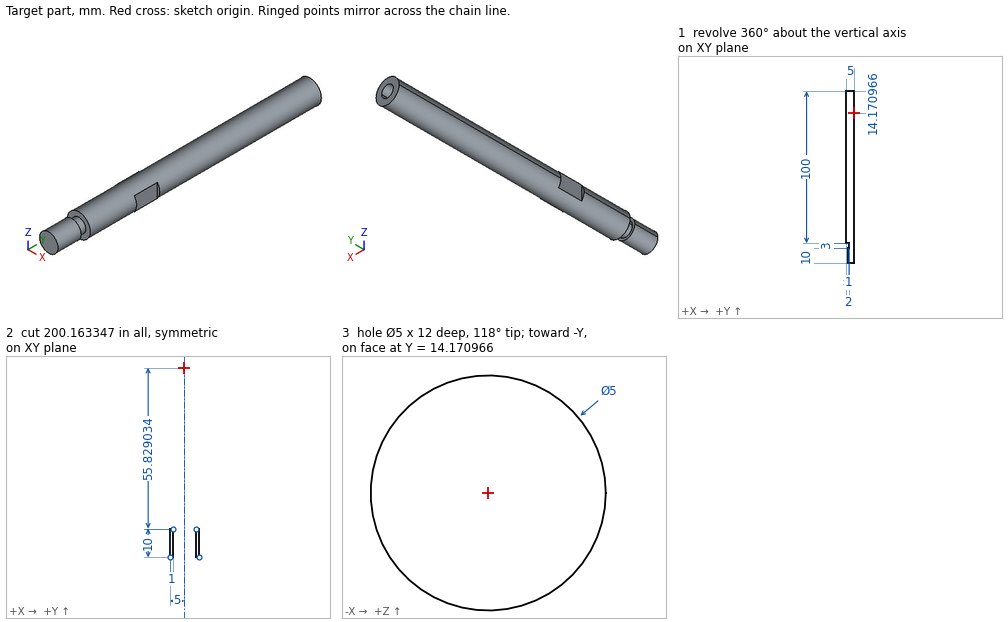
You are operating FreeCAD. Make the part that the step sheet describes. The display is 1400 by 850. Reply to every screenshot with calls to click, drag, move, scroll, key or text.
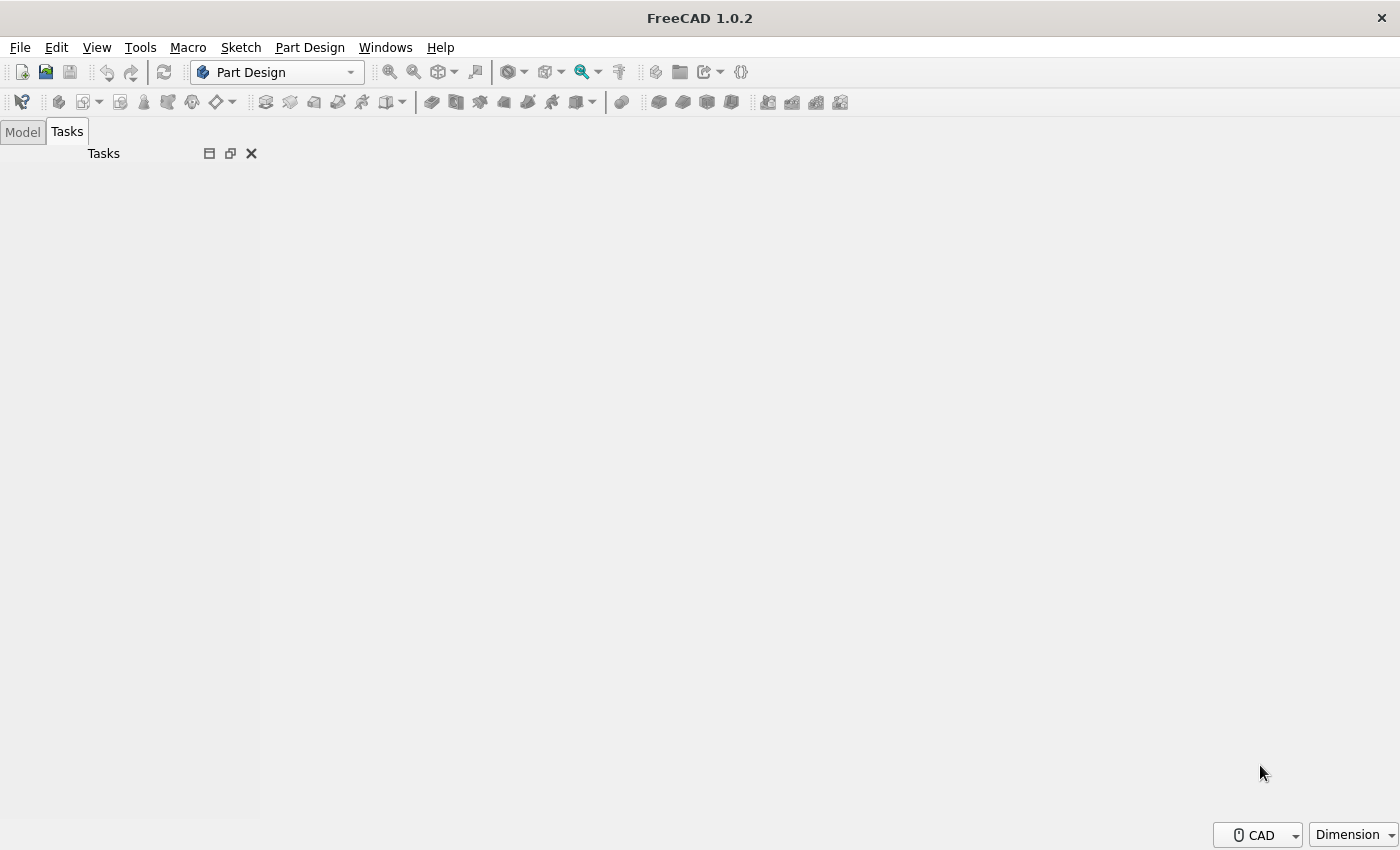
click(22, 72)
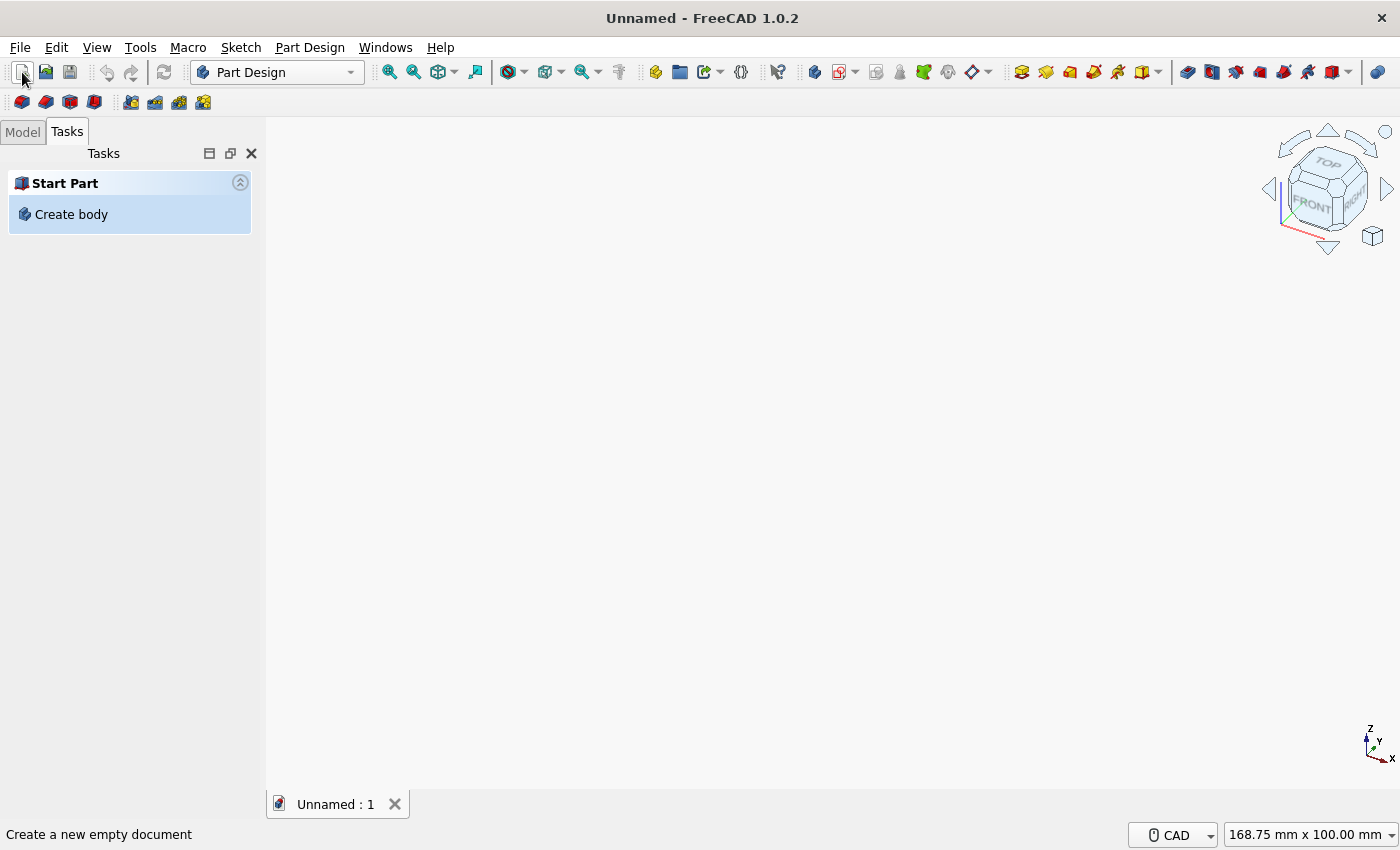
click(840, 72)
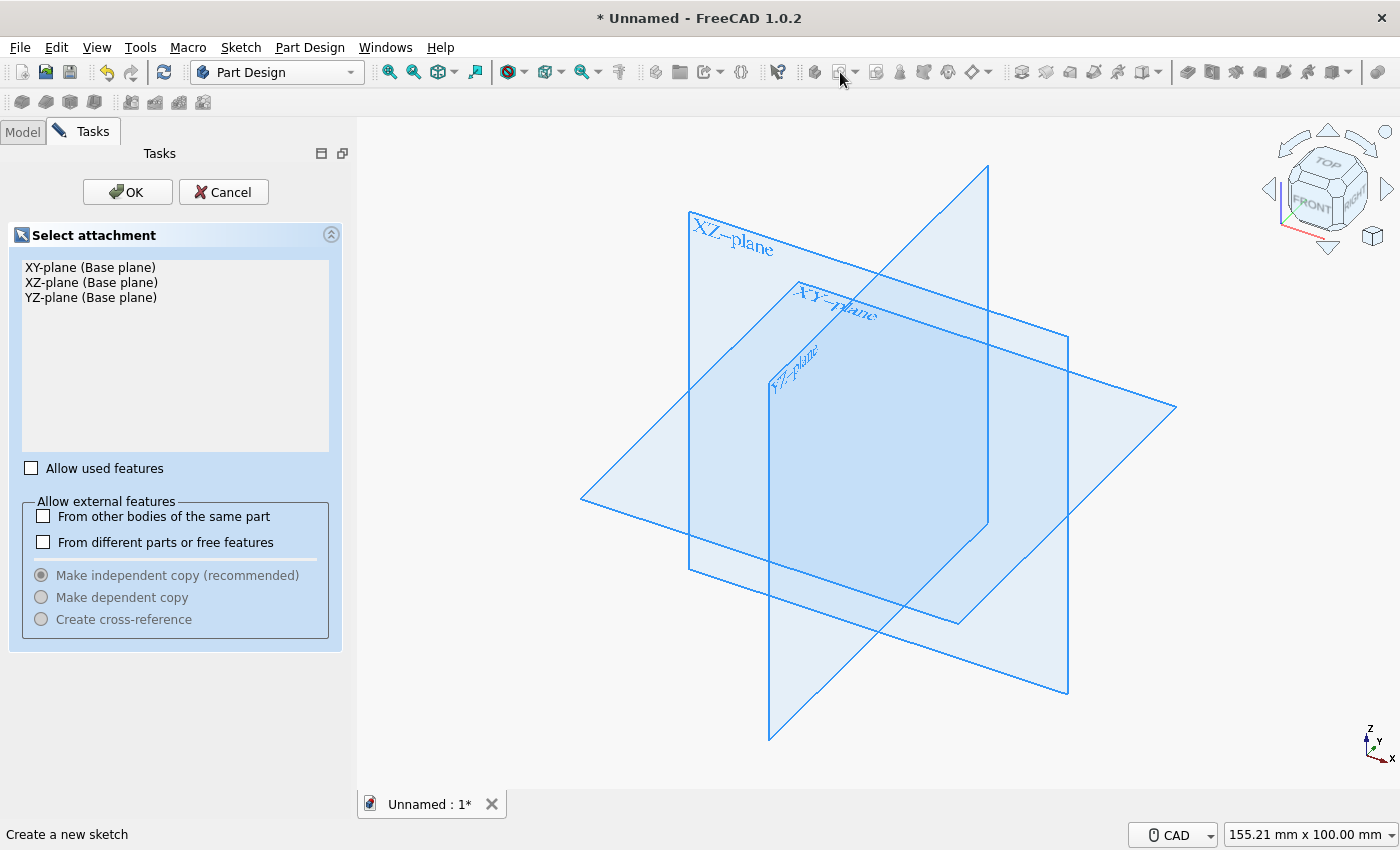
click(82, 268)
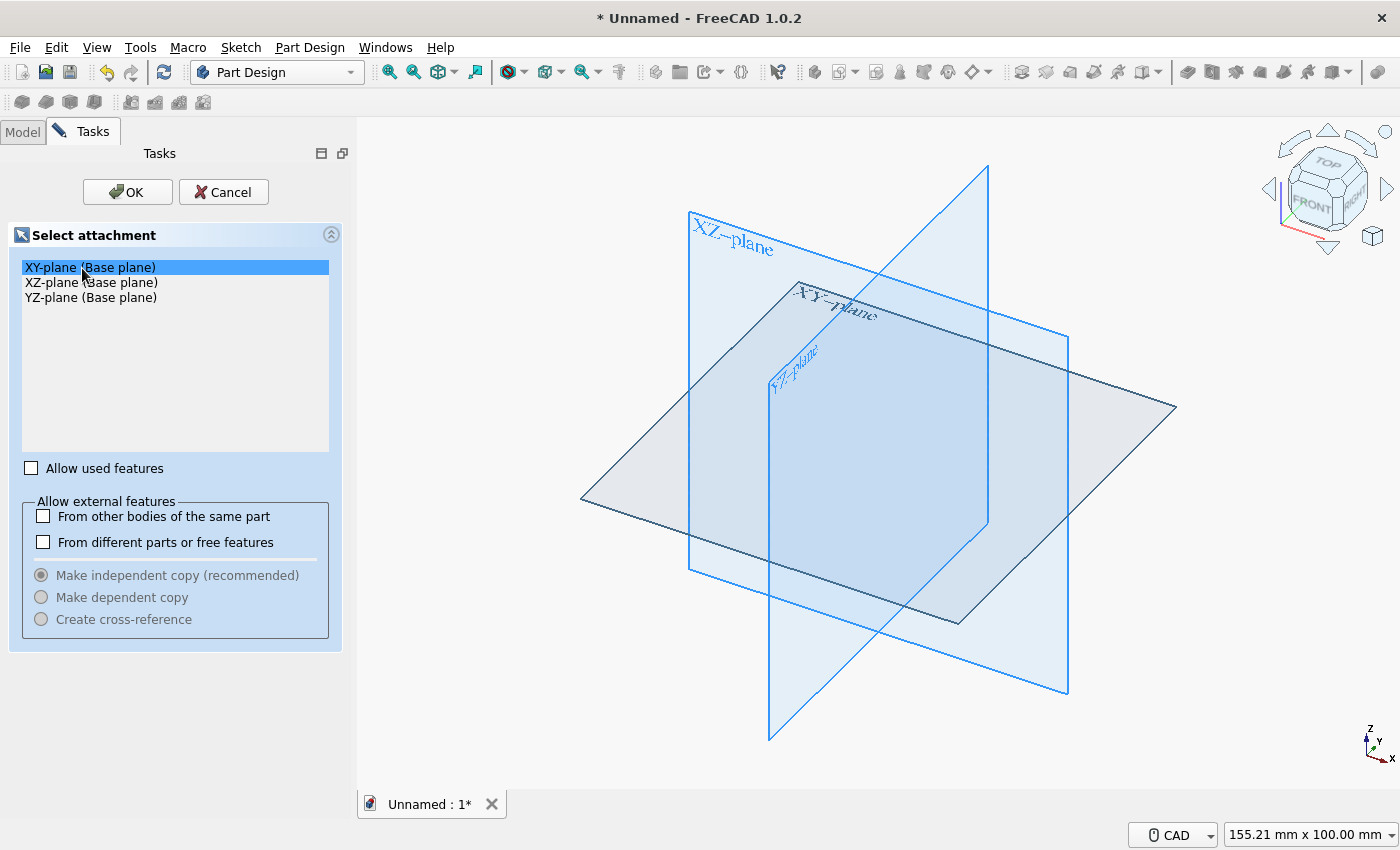
click(128, 192)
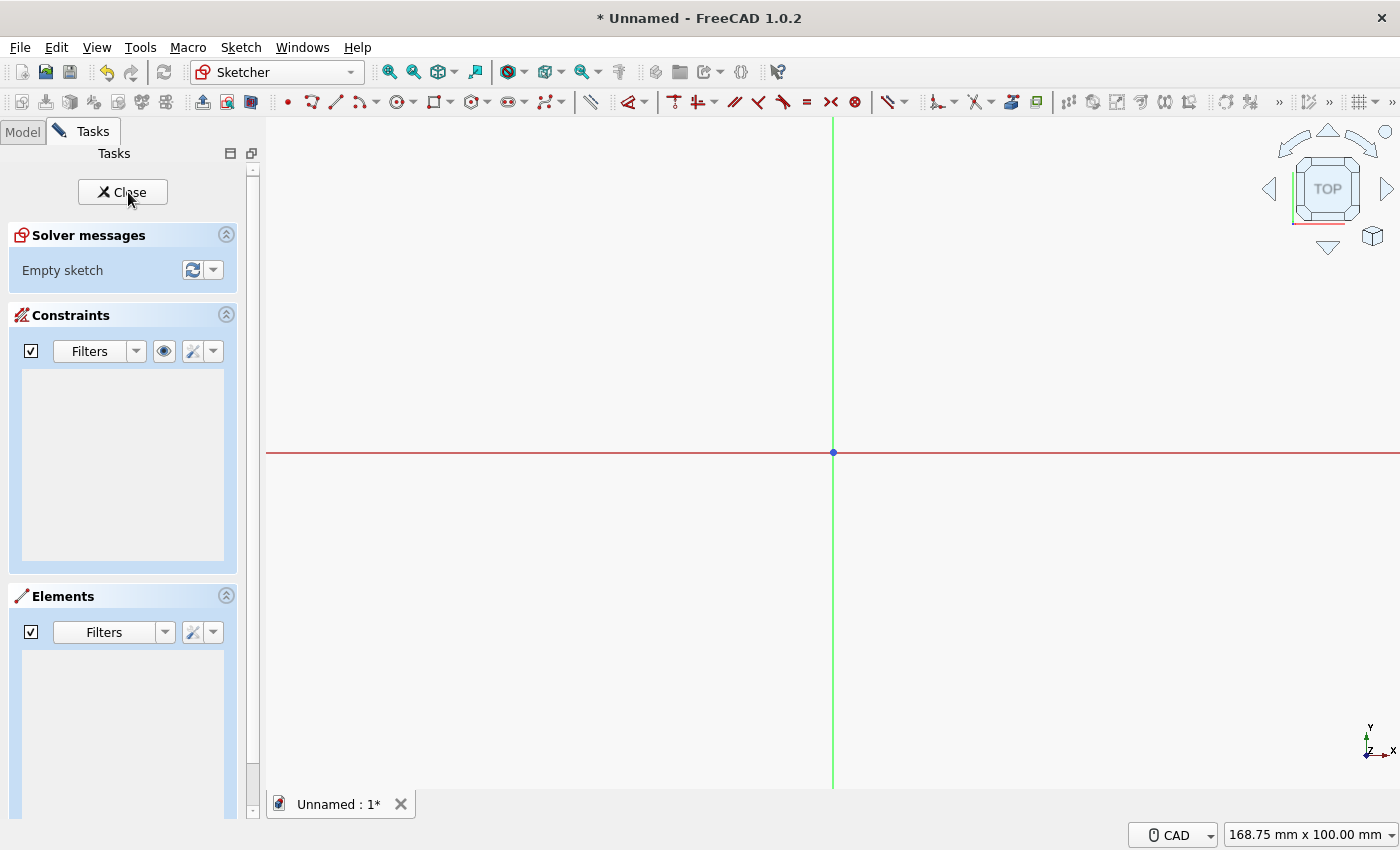
scroll(702, 145, down, 3)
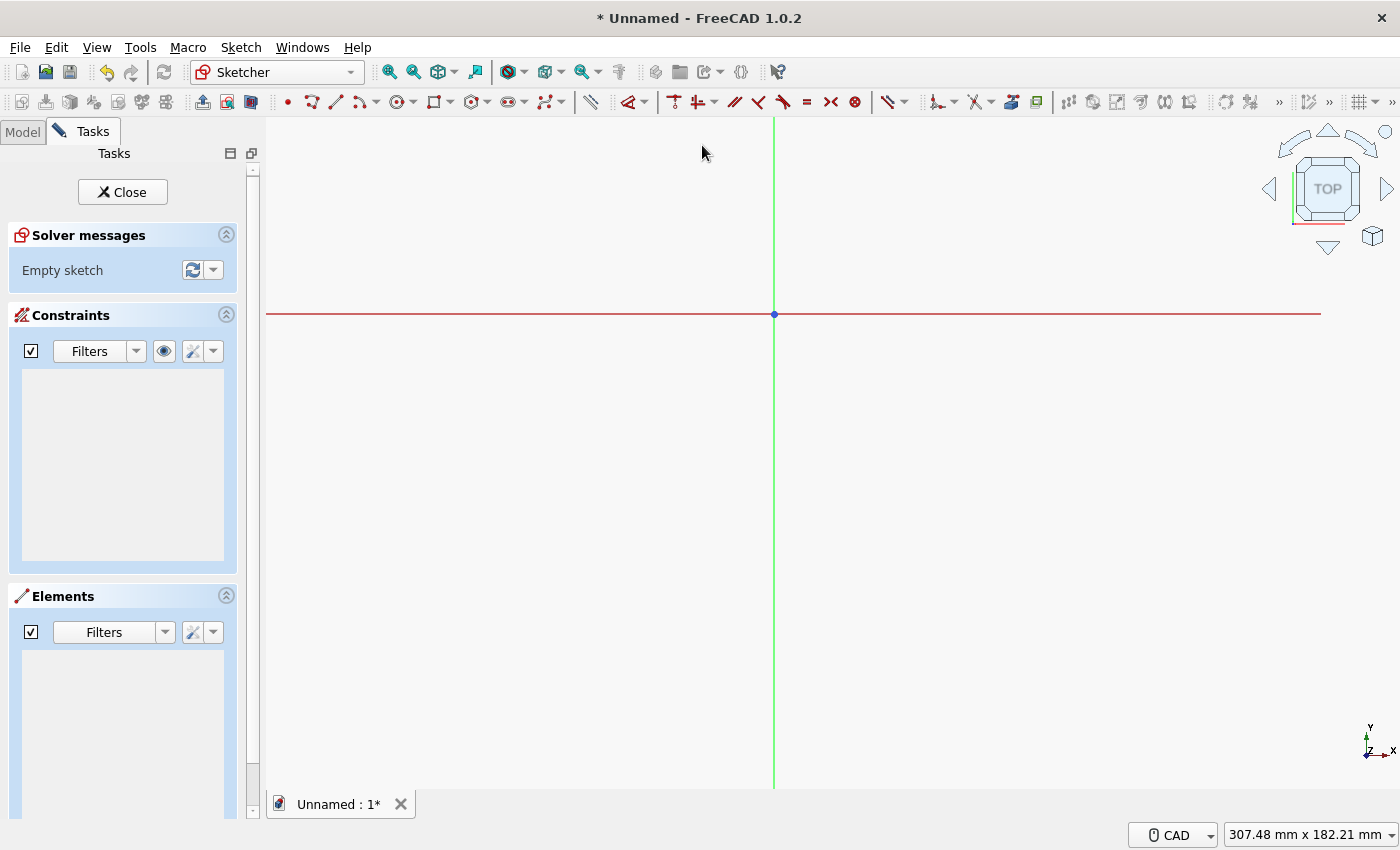
click(312, 102)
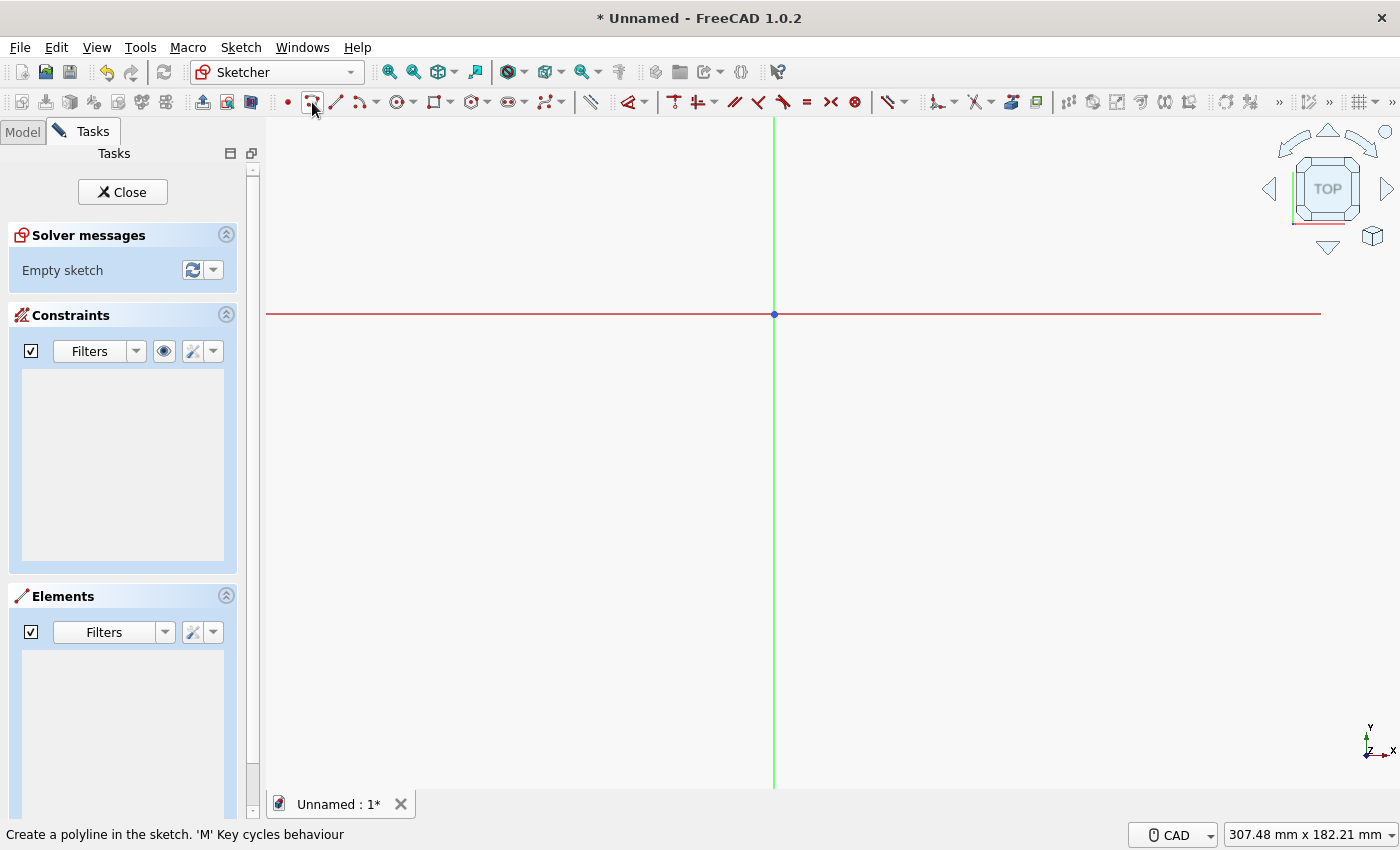
click(774, 262)
click(756, 262)
click(756, 631)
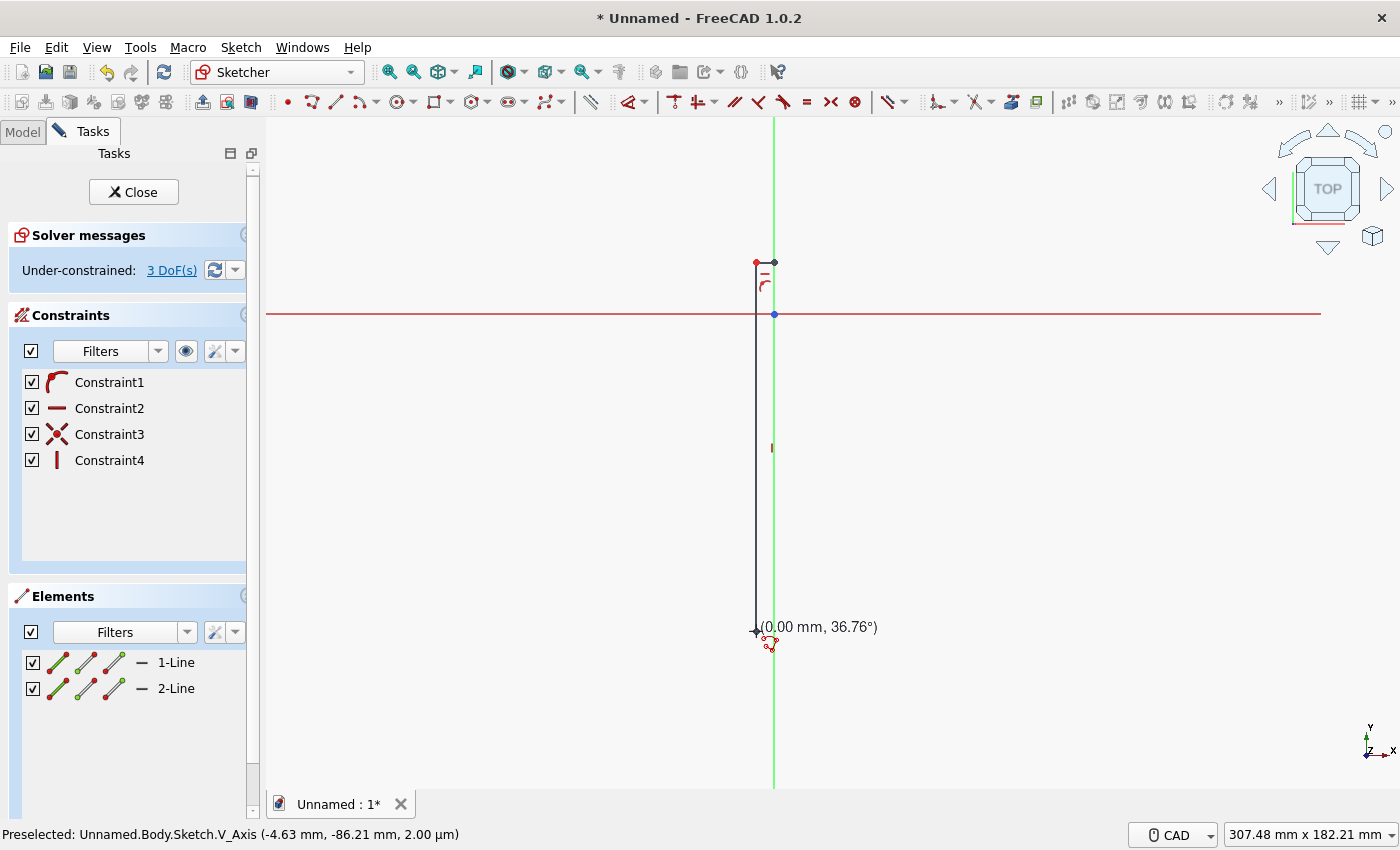
scroll(763, 631, up, 4)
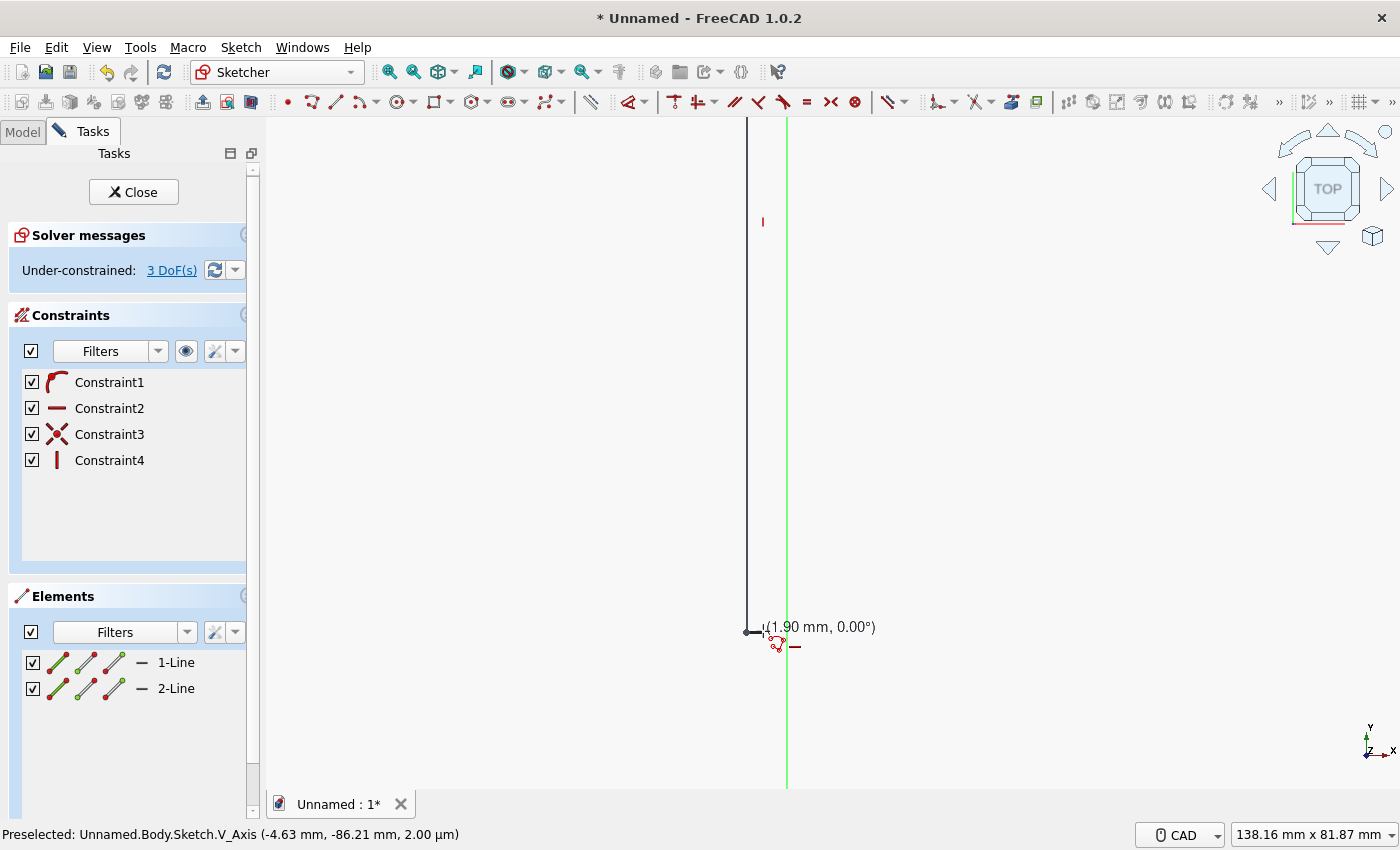
click(762, 630)
click(762, 654)